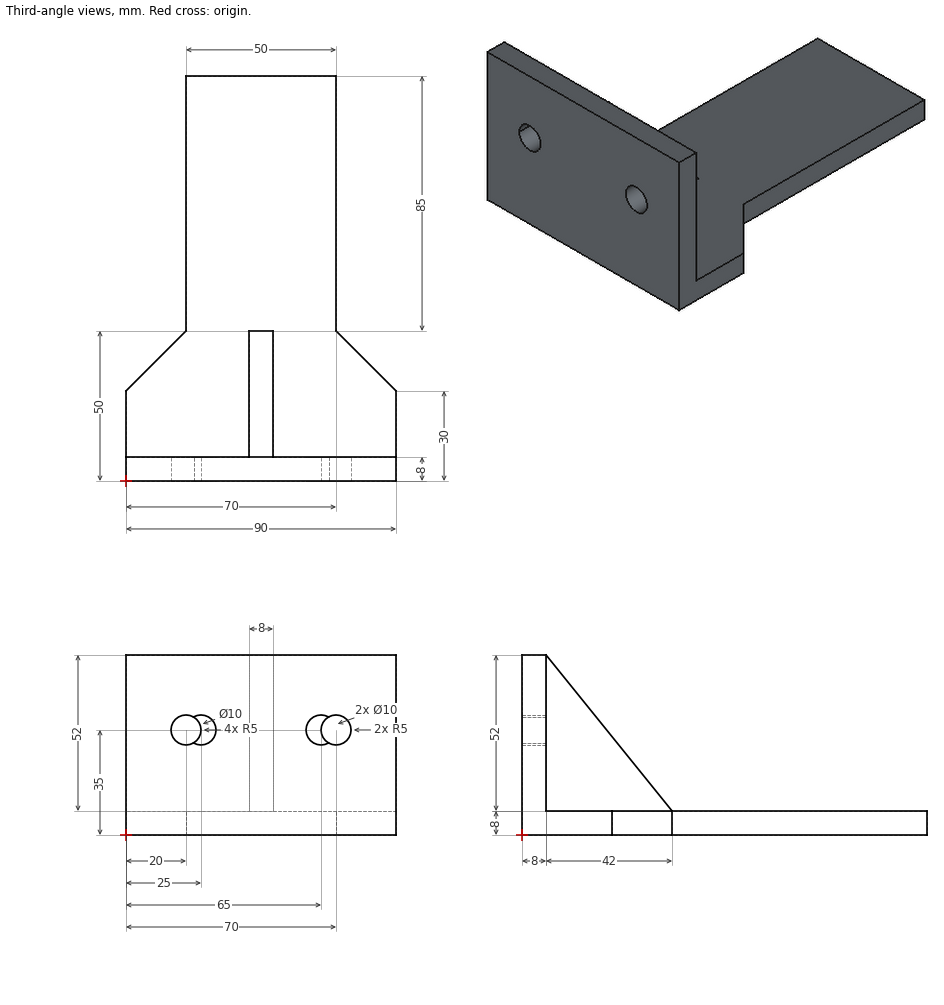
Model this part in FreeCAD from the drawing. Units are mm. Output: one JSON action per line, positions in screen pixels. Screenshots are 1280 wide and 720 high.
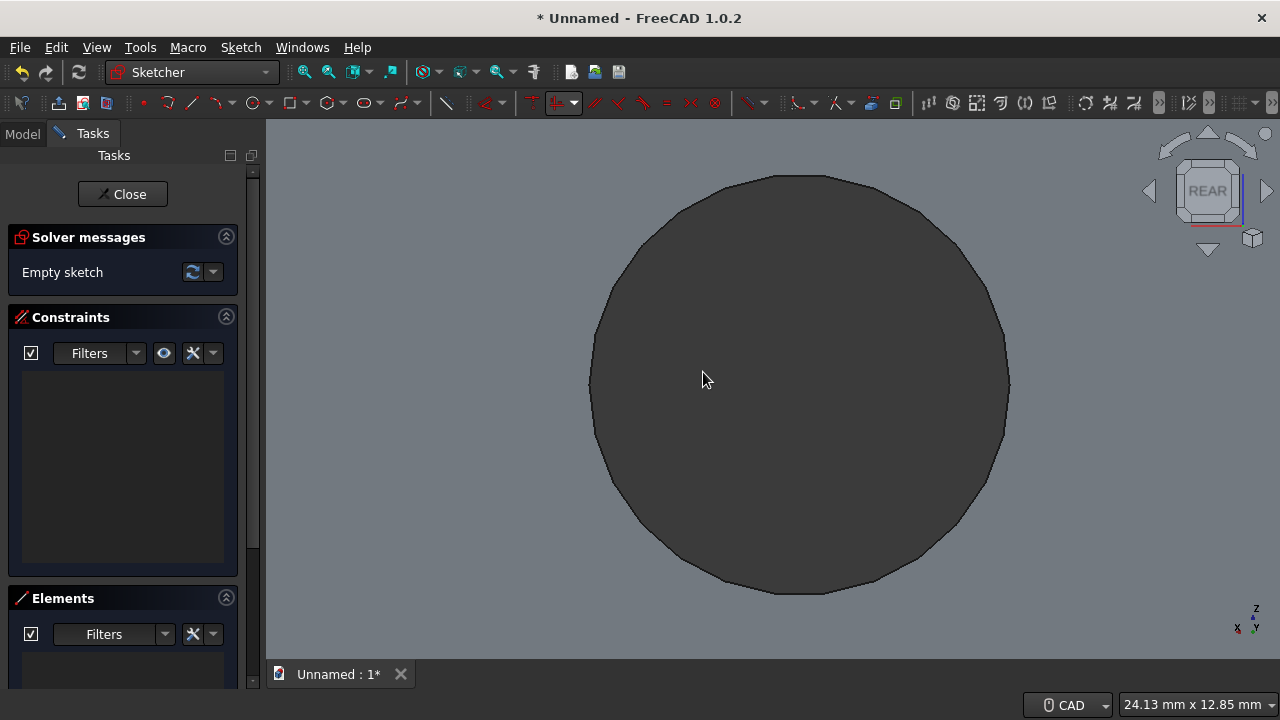
{"action": "left_click", "coordinate": [216, 104]}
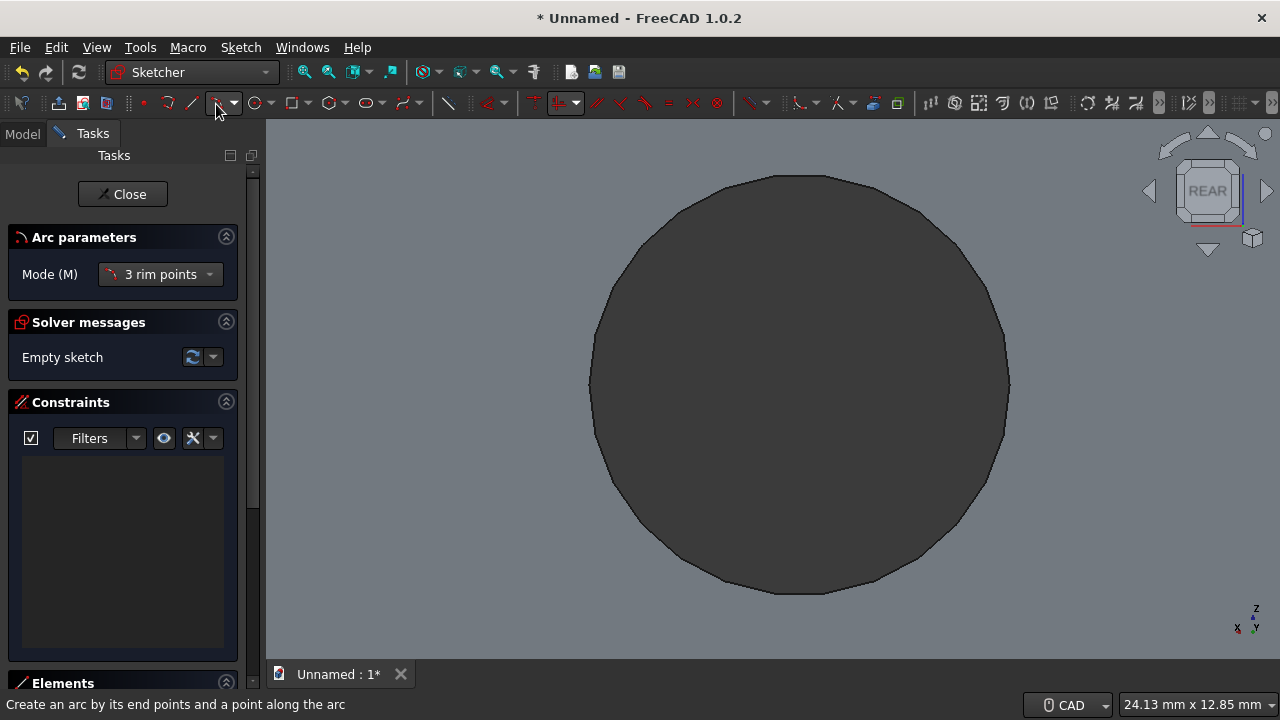
{"action": "left_click", "coordinate": [694, 567]}
{"action": "left_click", "coordinate": [694, 203]}
{"action": "left_click", "coordinate": [1010, 385]}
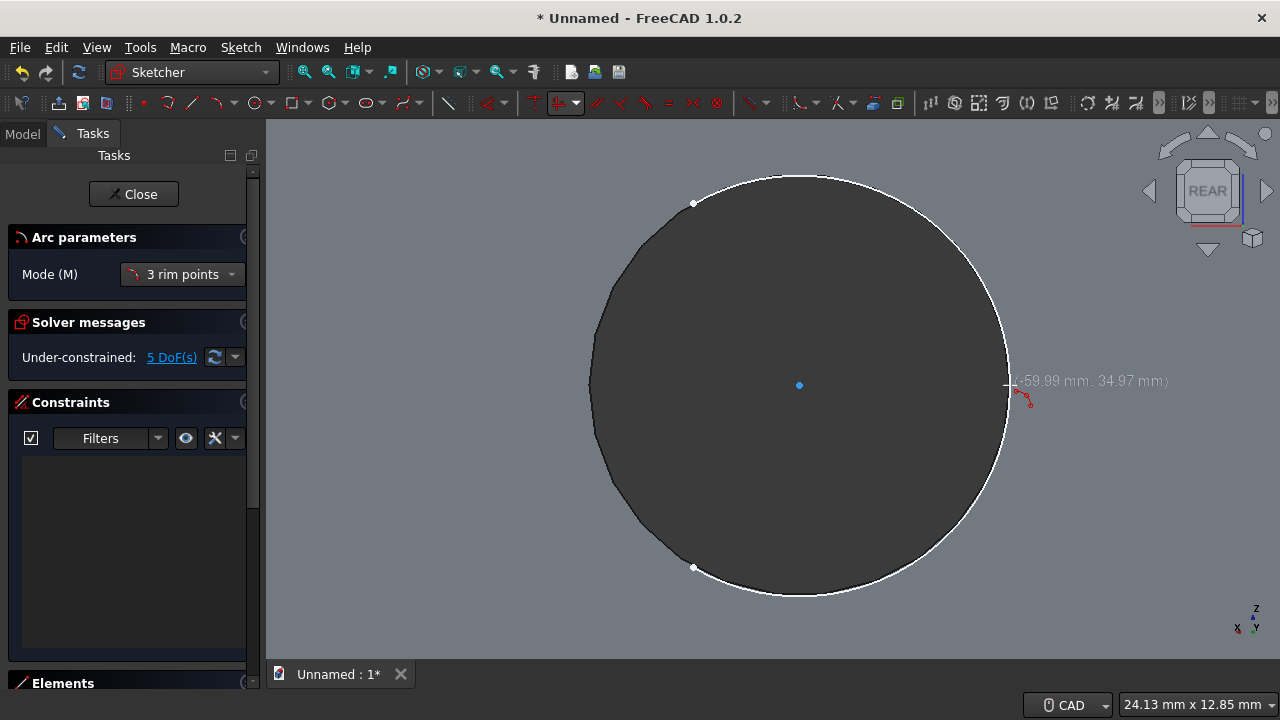
{"action": "left_click", "coordinate": [694, 204]}
{"action": "left_click", "coordinate": [694, 568]}
{"action": "left_click", "coordinate": [379, 385]}
{"action": "key", "text": "Escape"}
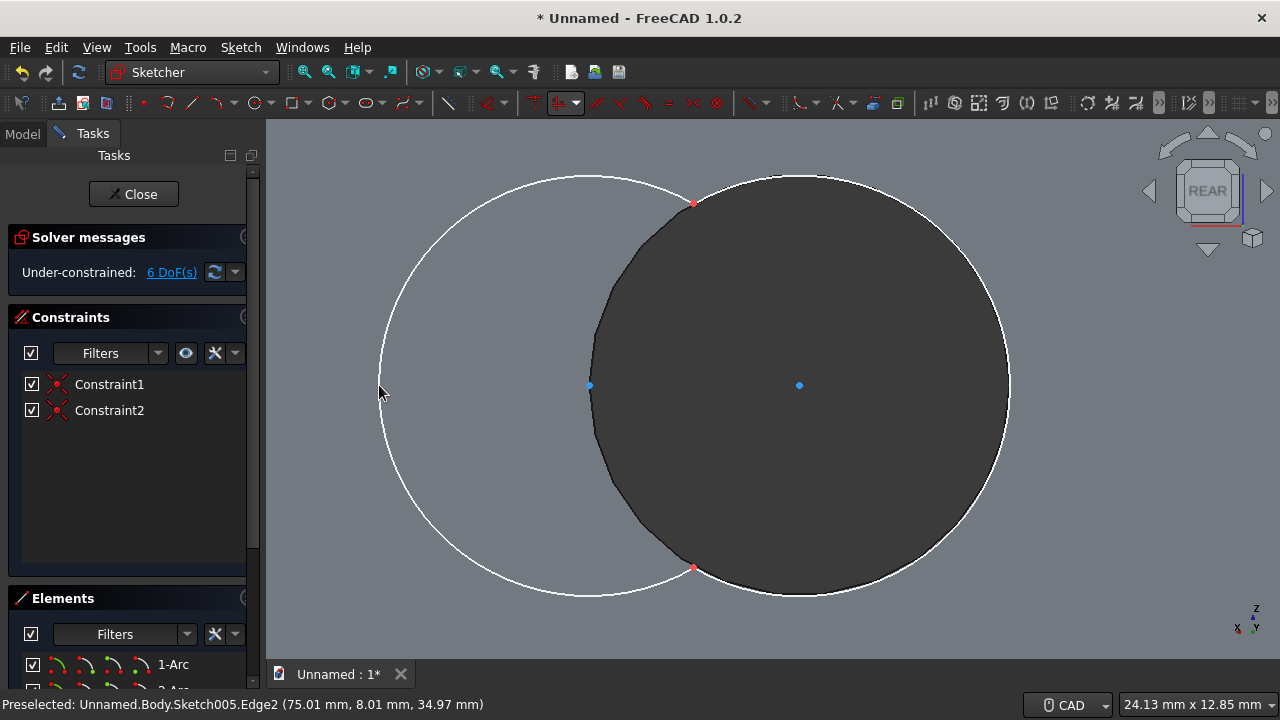
{"action": "left_click", "coordinate": [940, 542]}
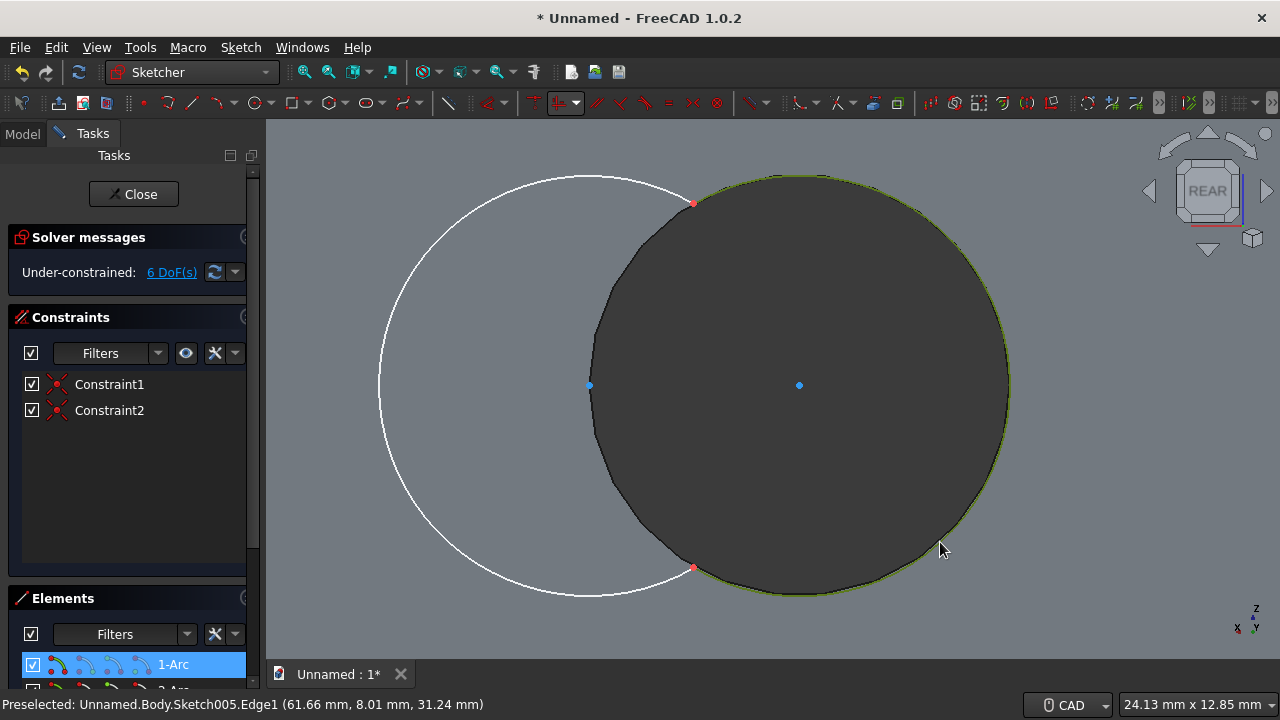
{"action": "left_click", "coordinate": [448, 230]}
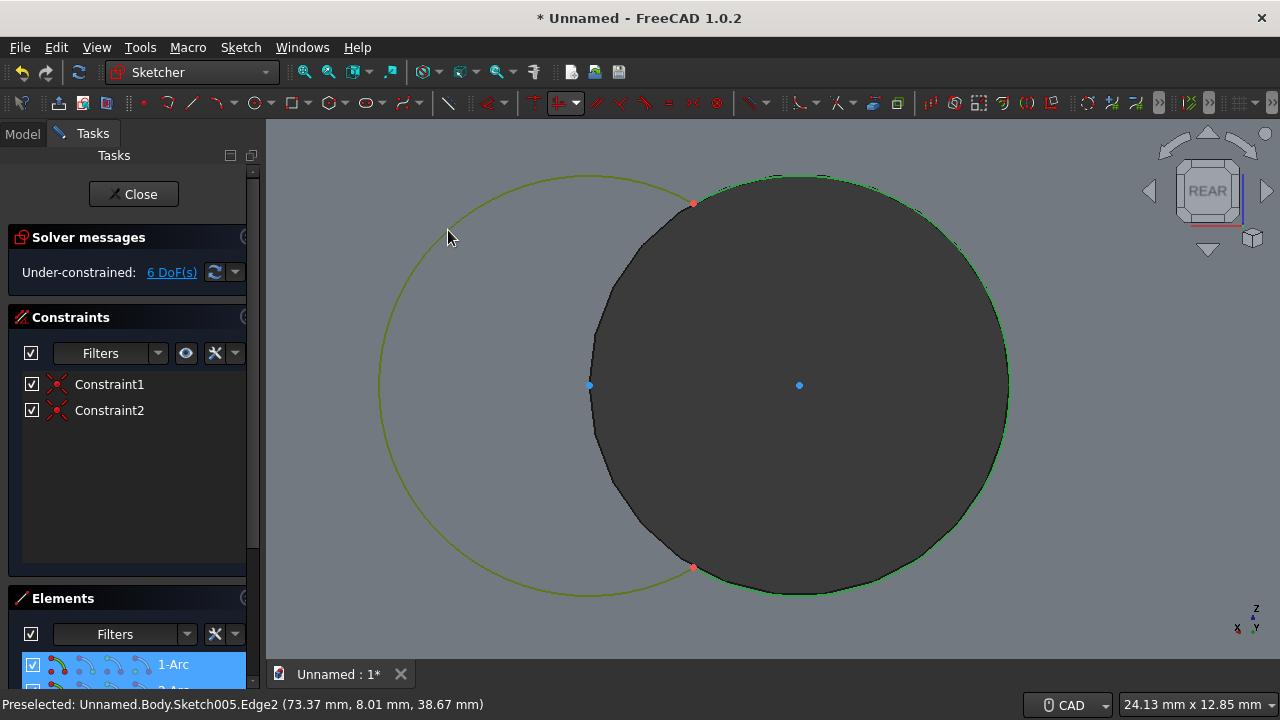
{"action": "left_click", "coordinate": [670, 104]}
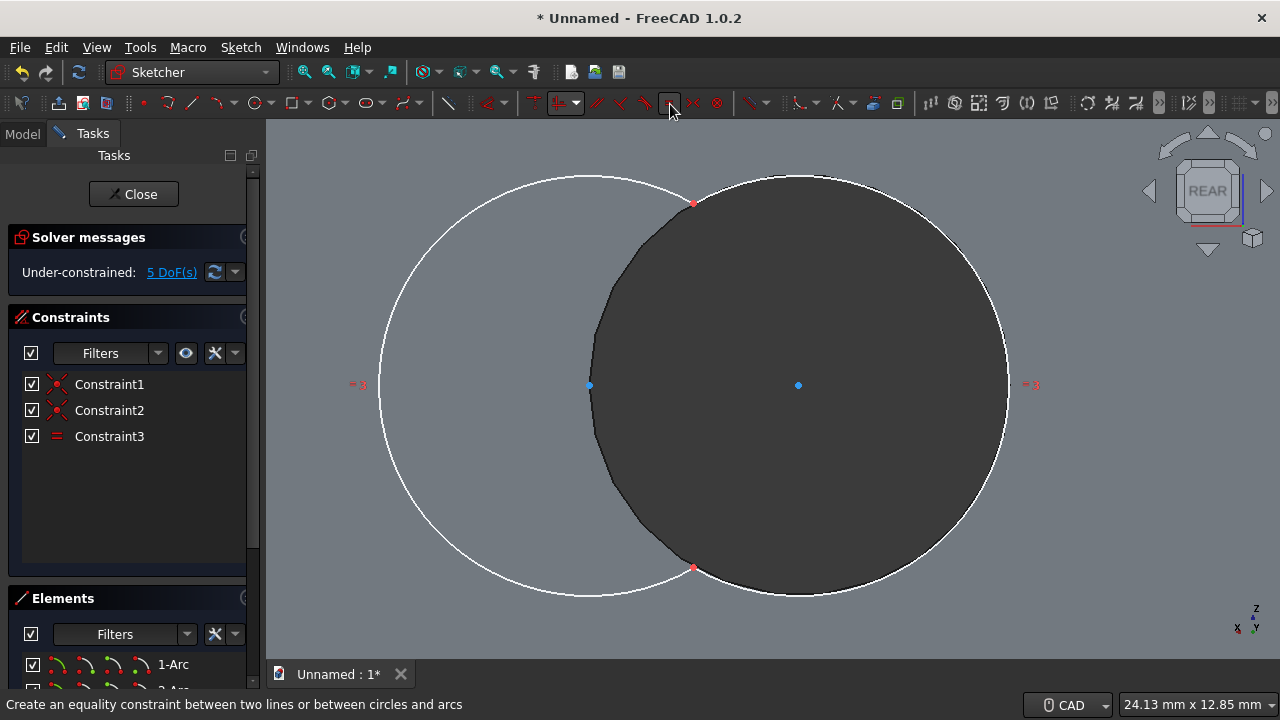
{"action": "left_click", "coordinate": [488, 104]}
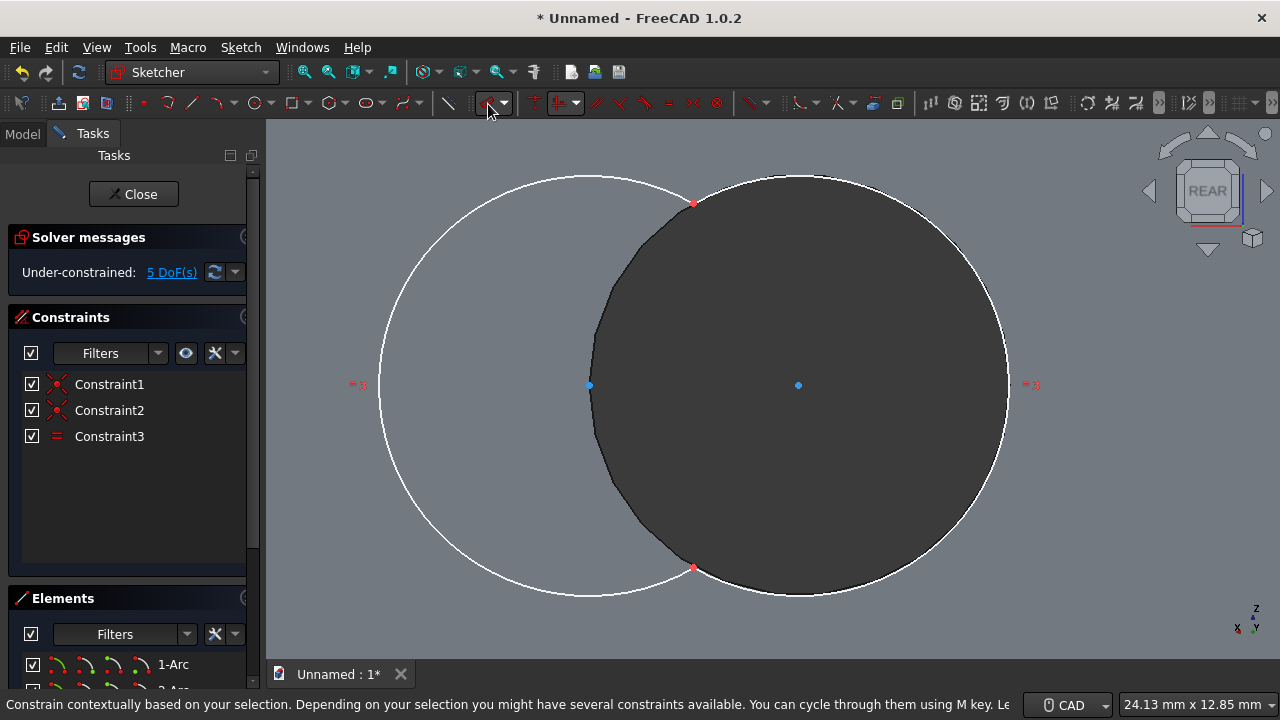
{"action": "left_click", "coordinate": [940, 542]}
{"action": "left_click", "coordinate": [961, 566]}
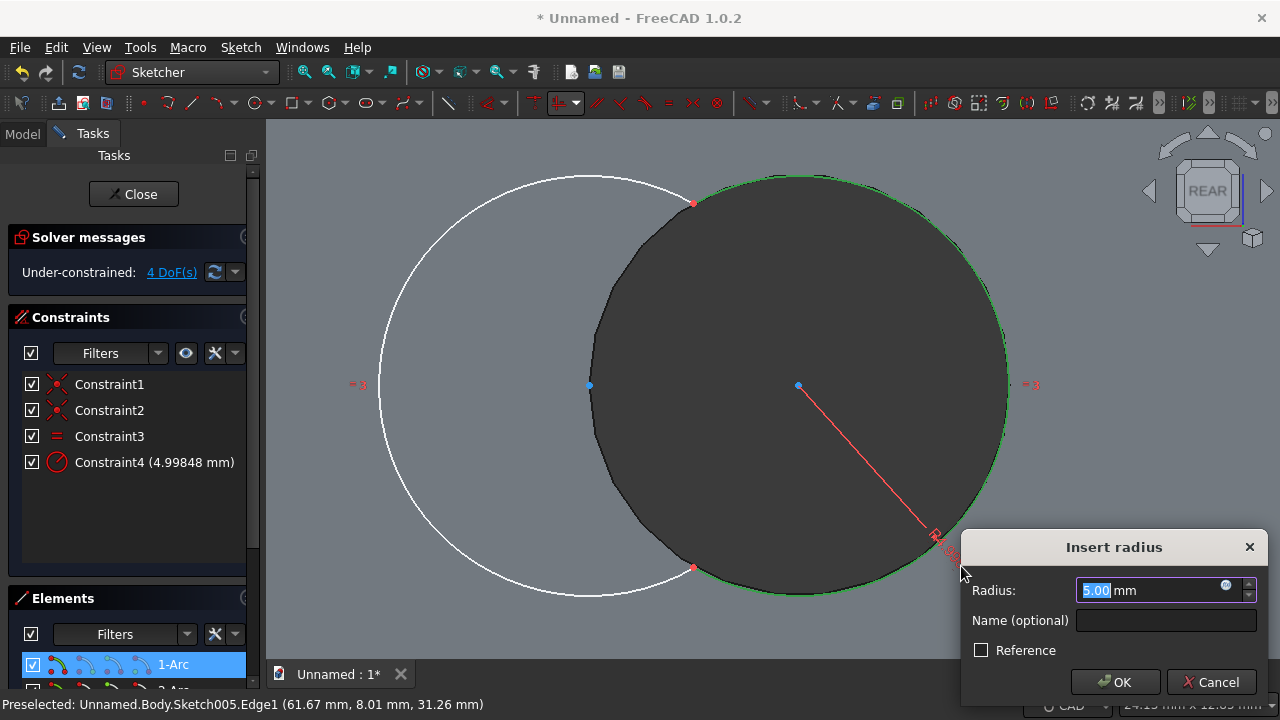
{"action": "type", "text": "5"}
{"action": "key", "text": "Return"}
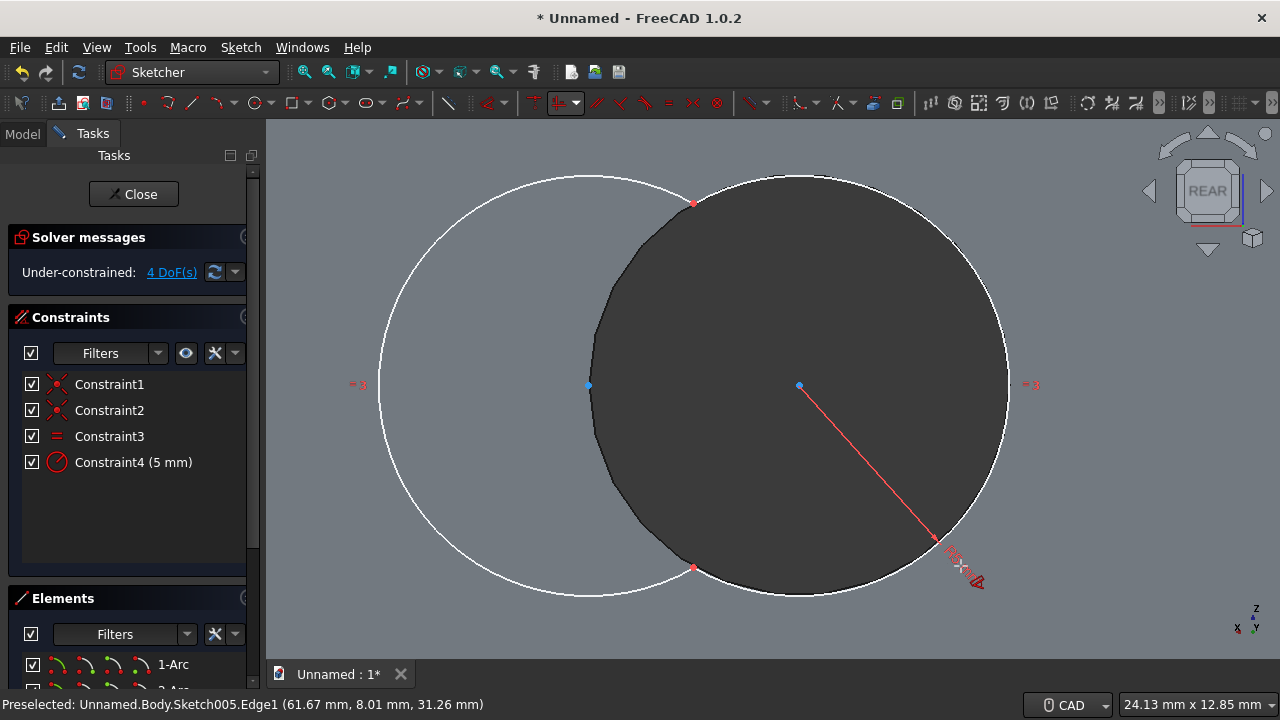
{"action": "left_click", "coordinate": [799, 386]}
{"action": "left_click", "coordinate": [957, 352]}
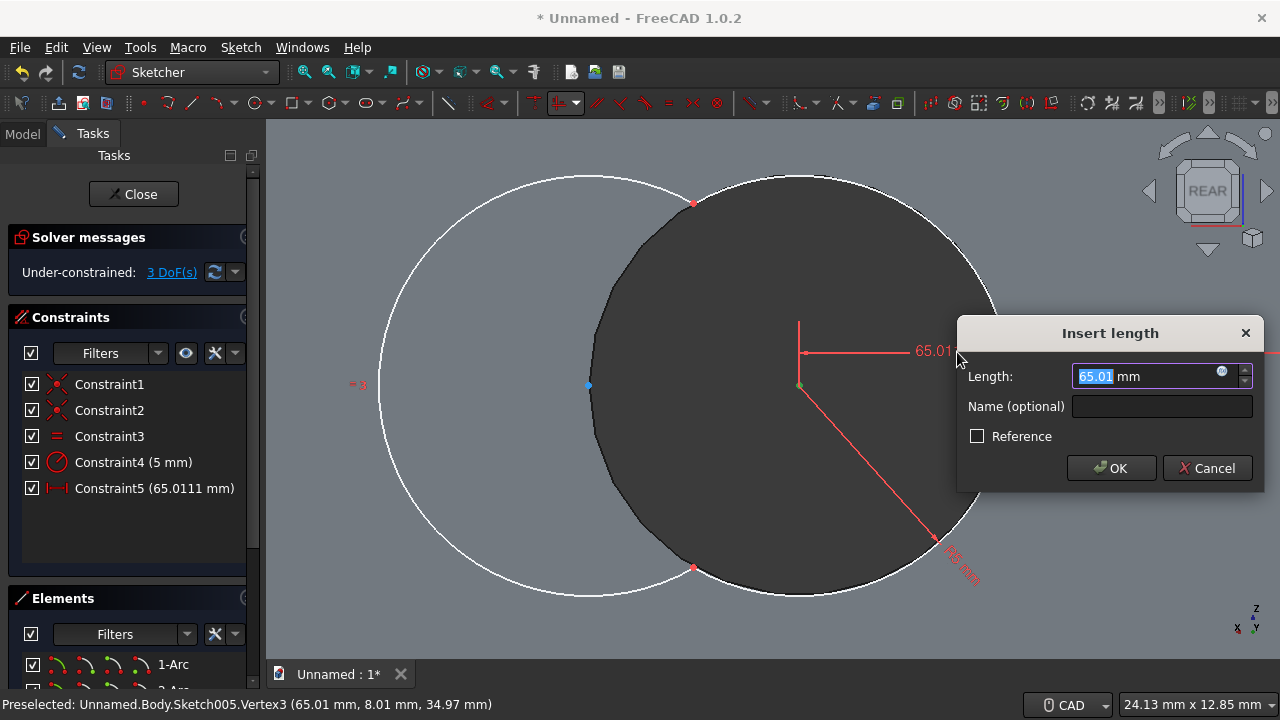
{"action": "type", "text": "65"}
{"action": "key", "text": "Return"}